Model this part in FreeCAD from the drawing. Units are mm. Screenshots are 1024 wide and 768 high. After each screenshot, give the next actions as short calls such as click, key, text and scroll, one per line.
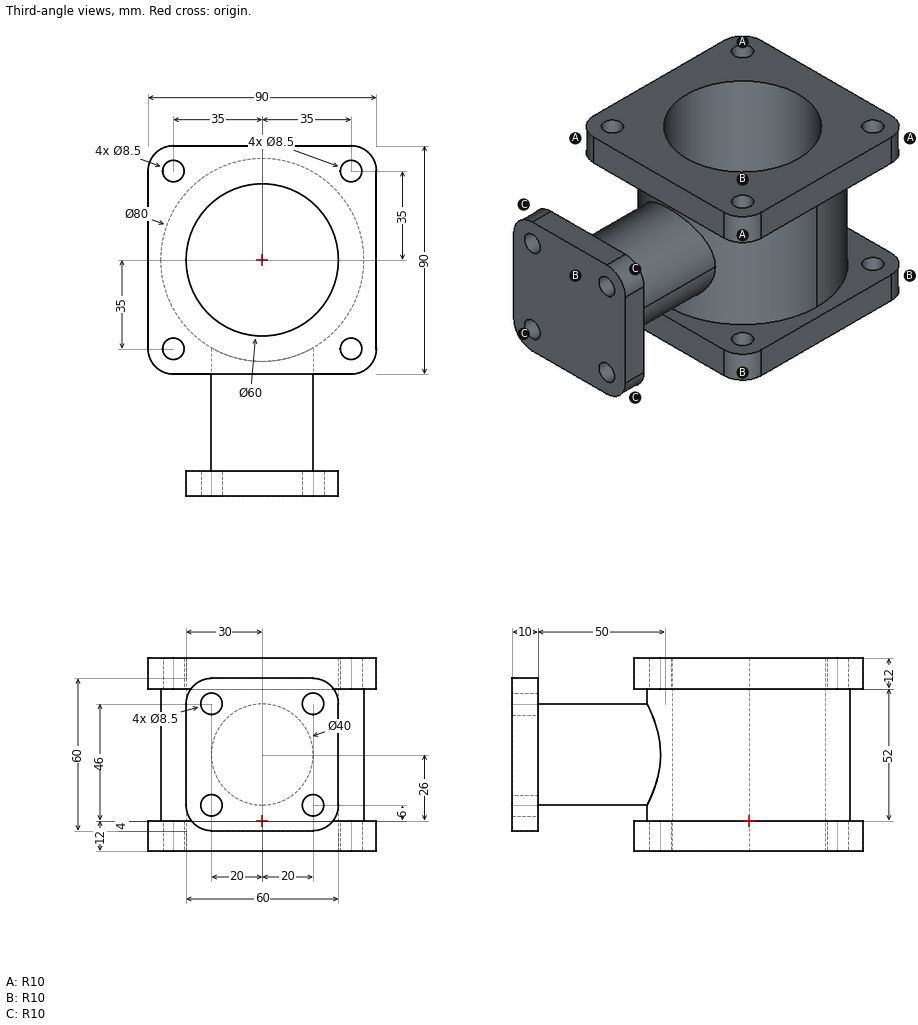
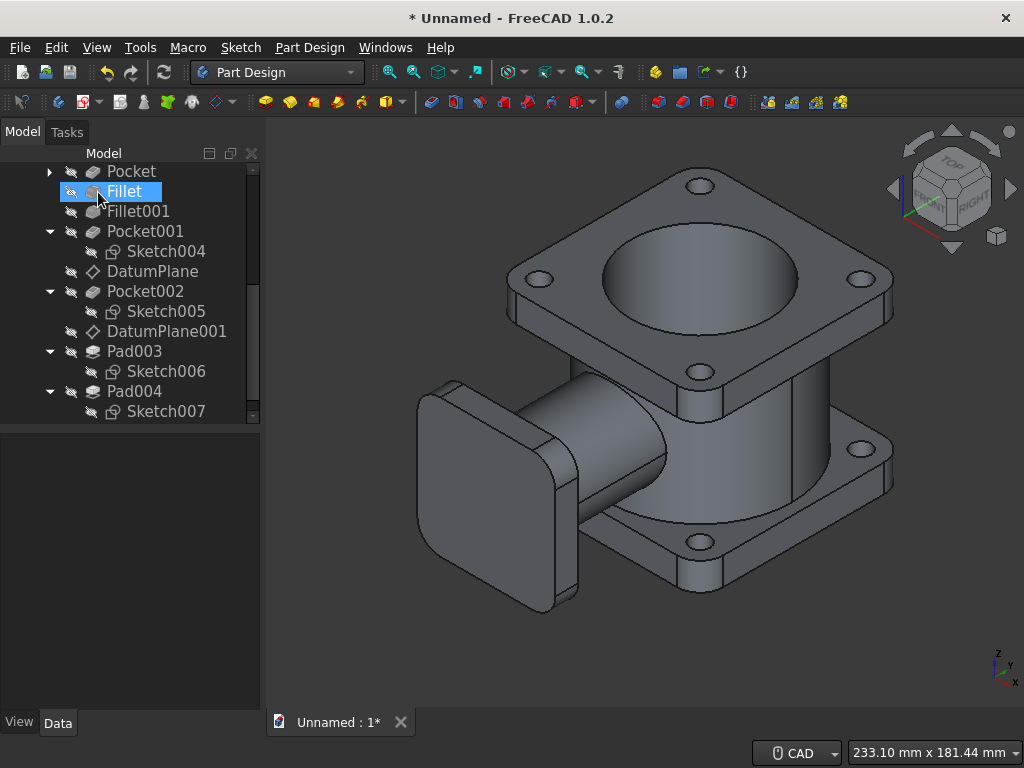
click(486, 503)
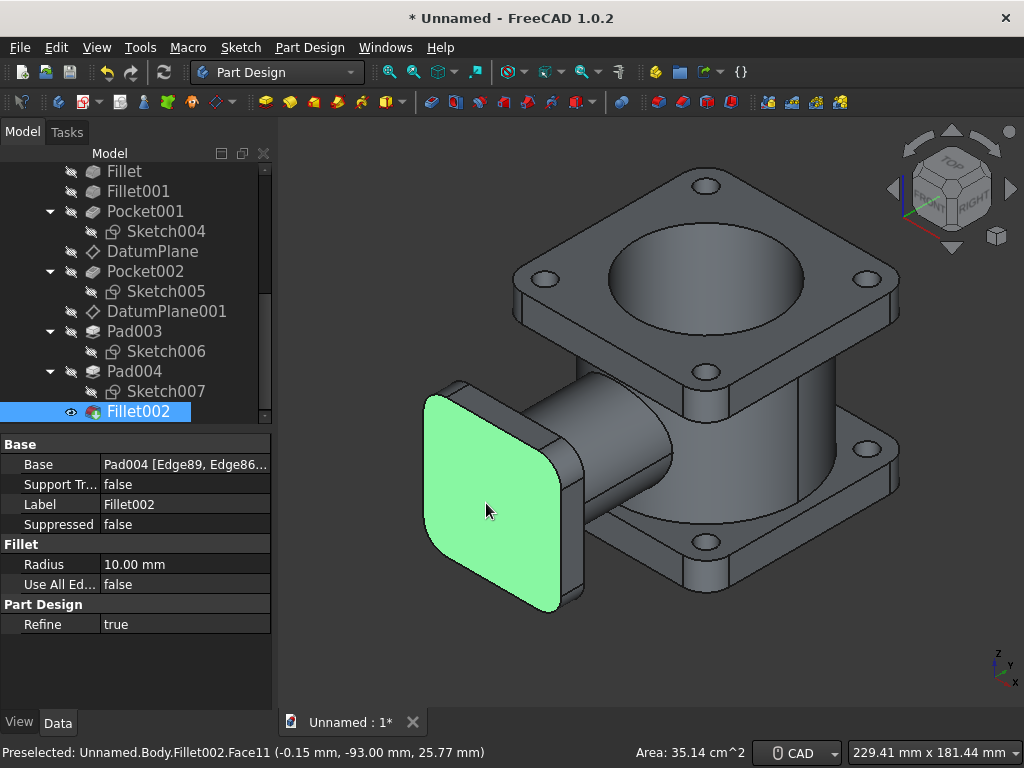
click(84, 102)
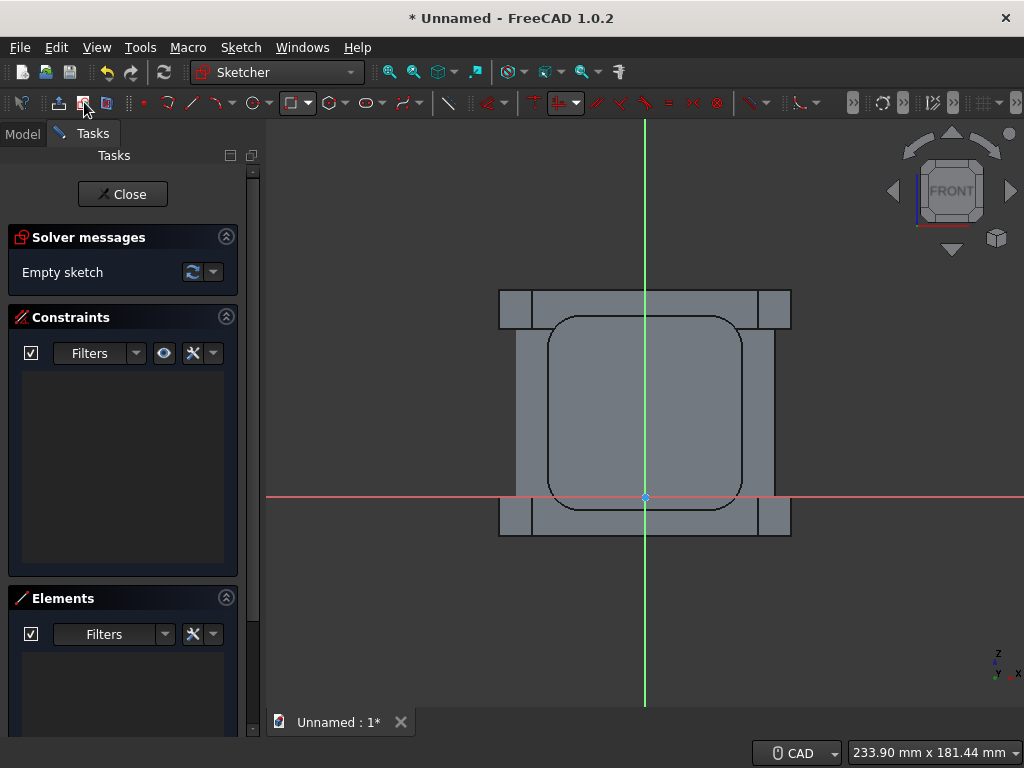
scroll(701, 418, up, 4)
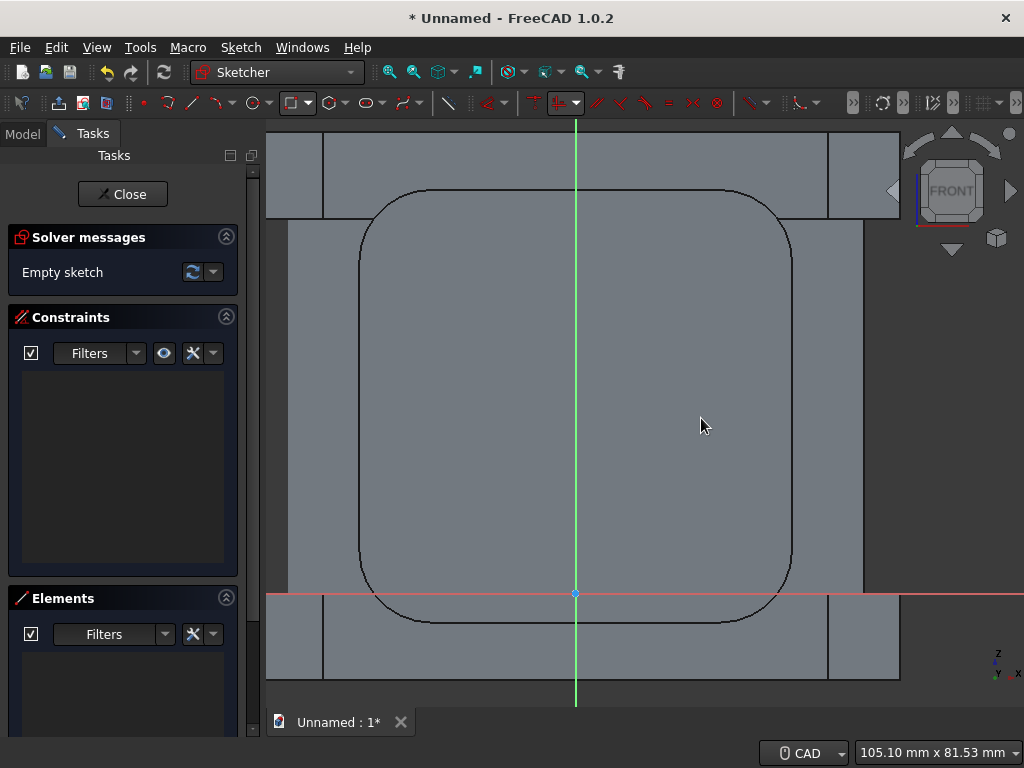
click(254, 104)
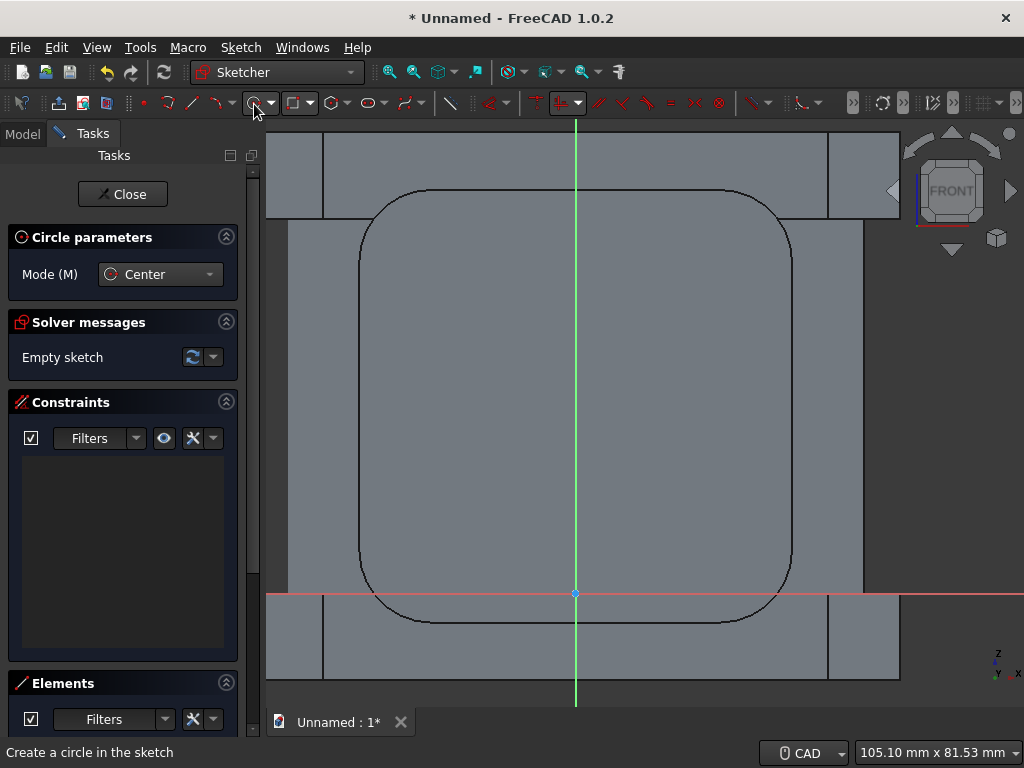
click(431, 262)
click(453, 240)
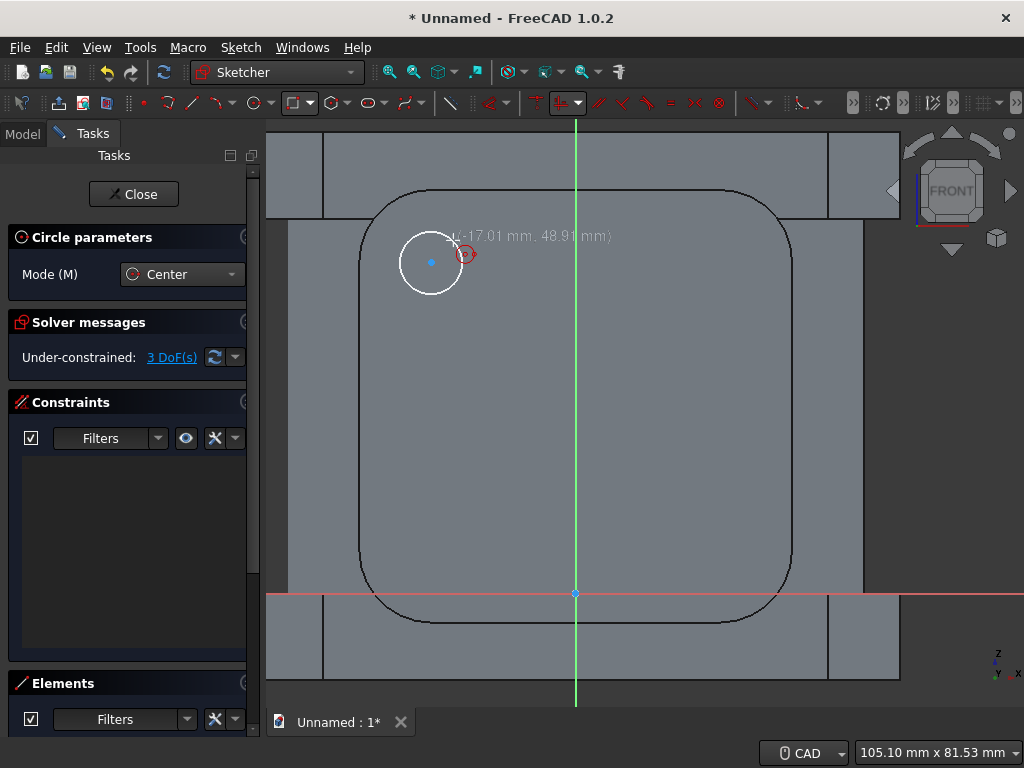
click(720, 262)
click(742, 240)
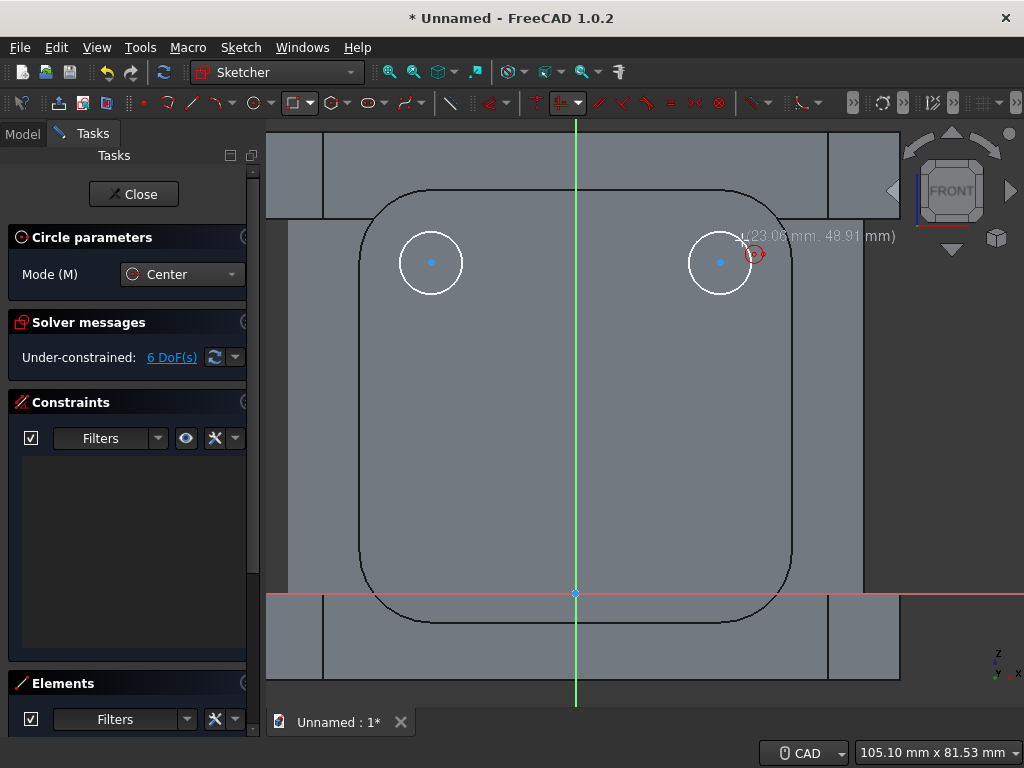
click(720, 550)
click(742, 529)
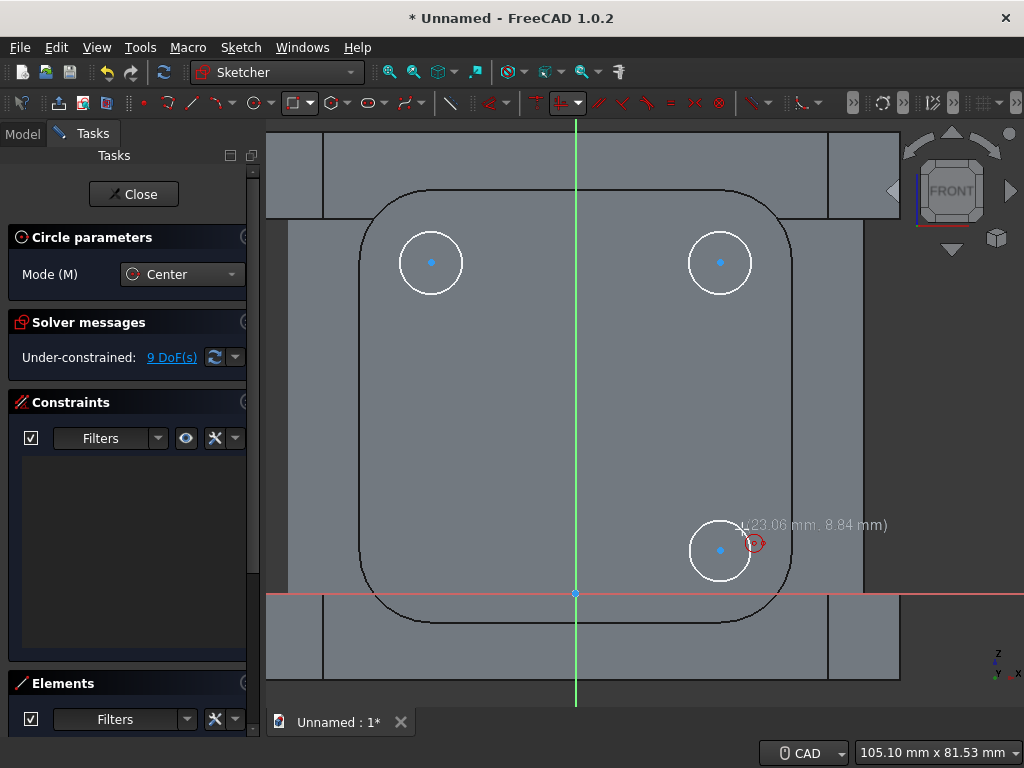
click(431, 550)
click(453, 529)
key(Escape)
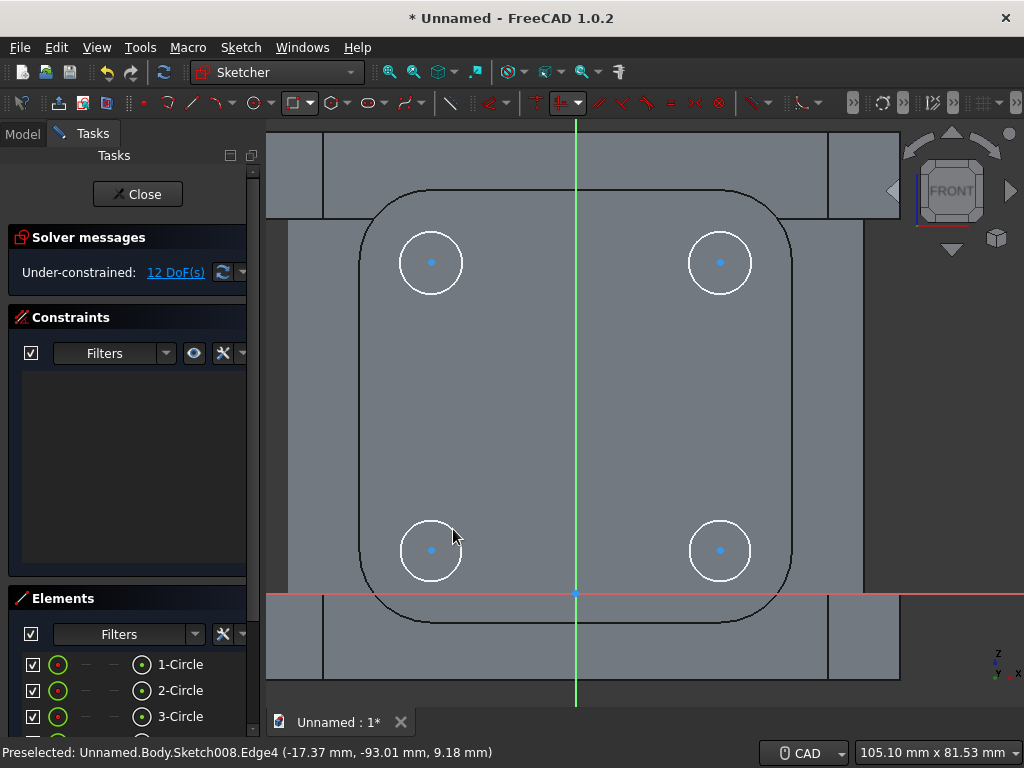
click(453, 241)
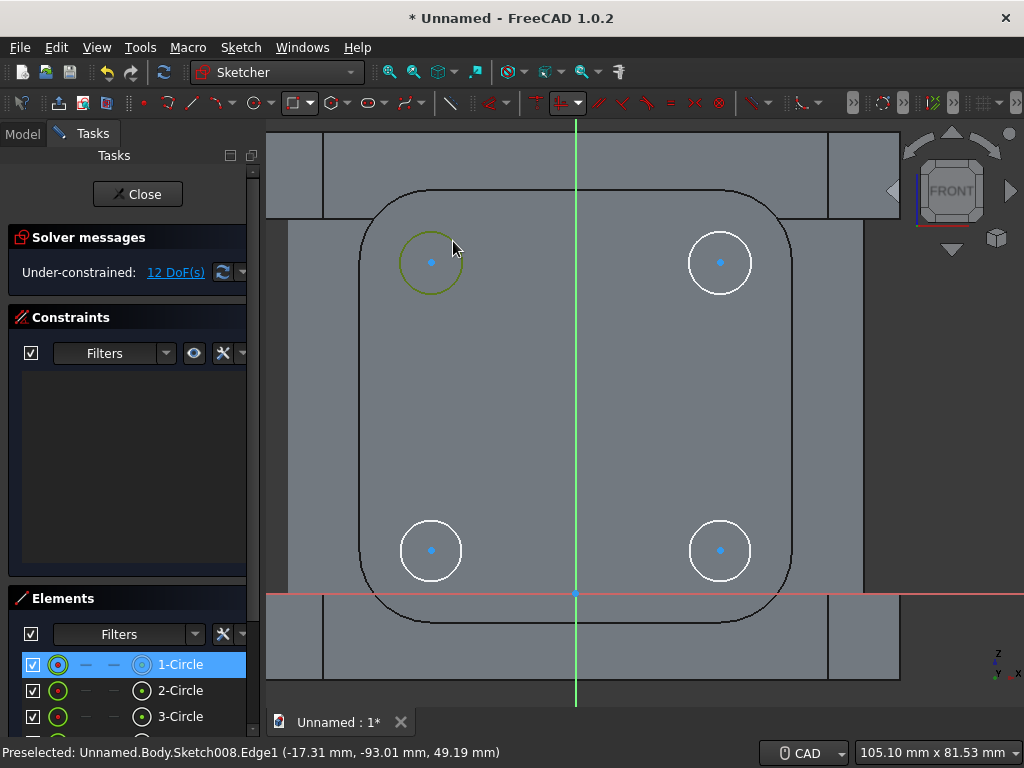
click(742, 241)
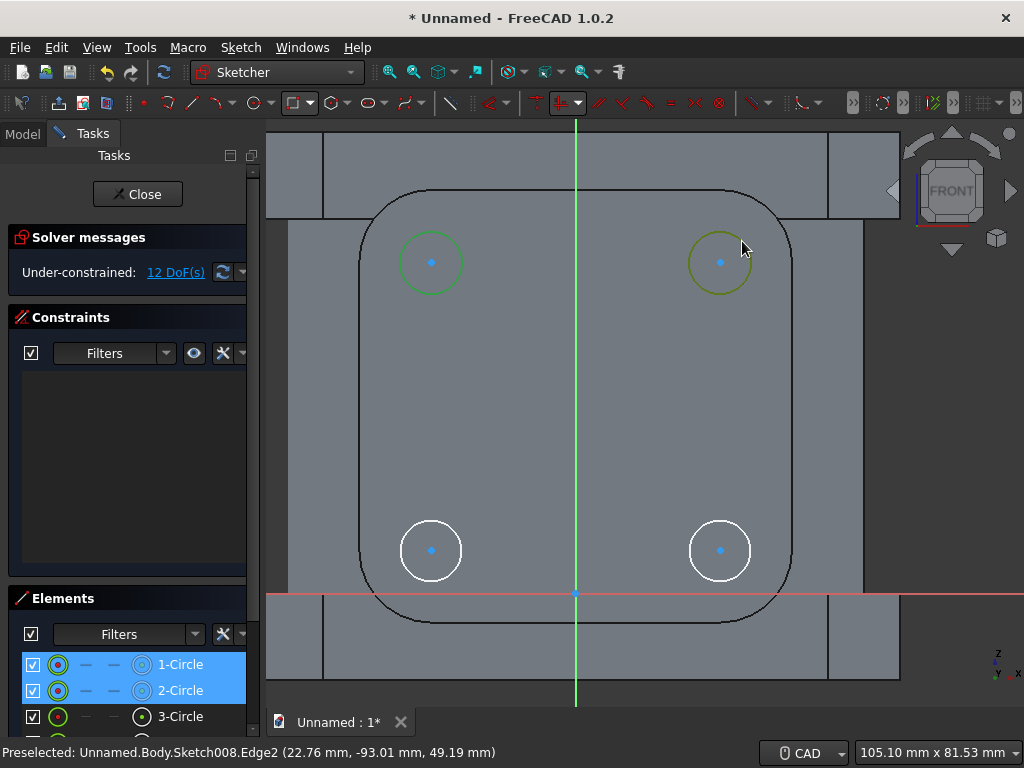
click(741, 529)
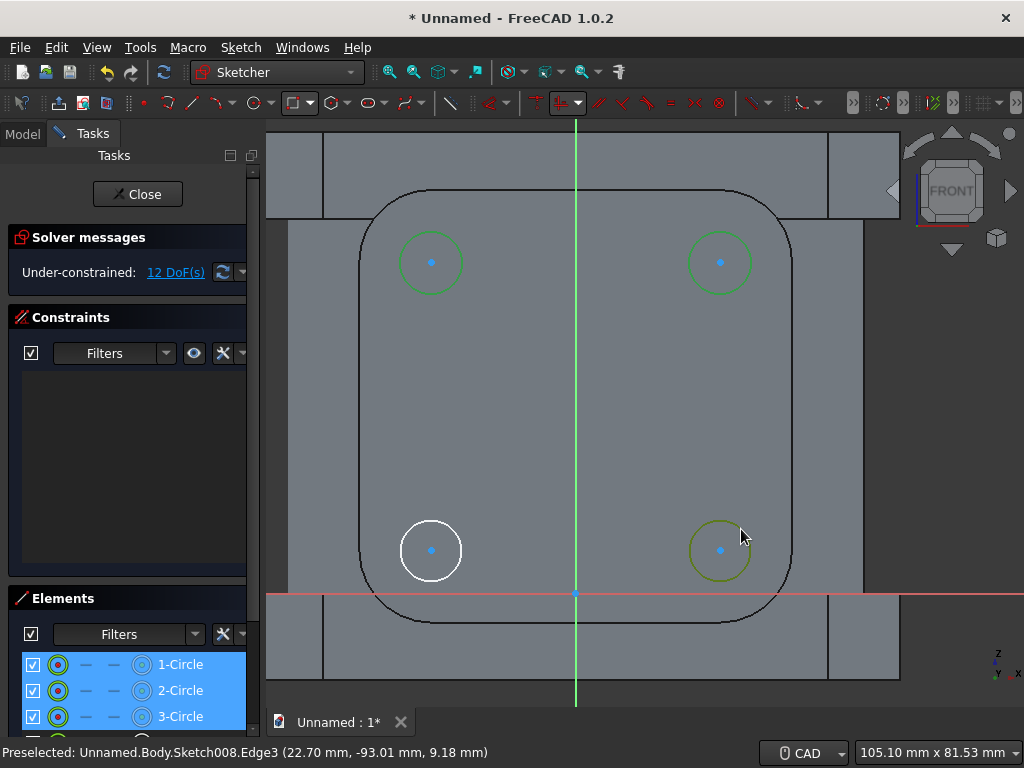
click(452, 529)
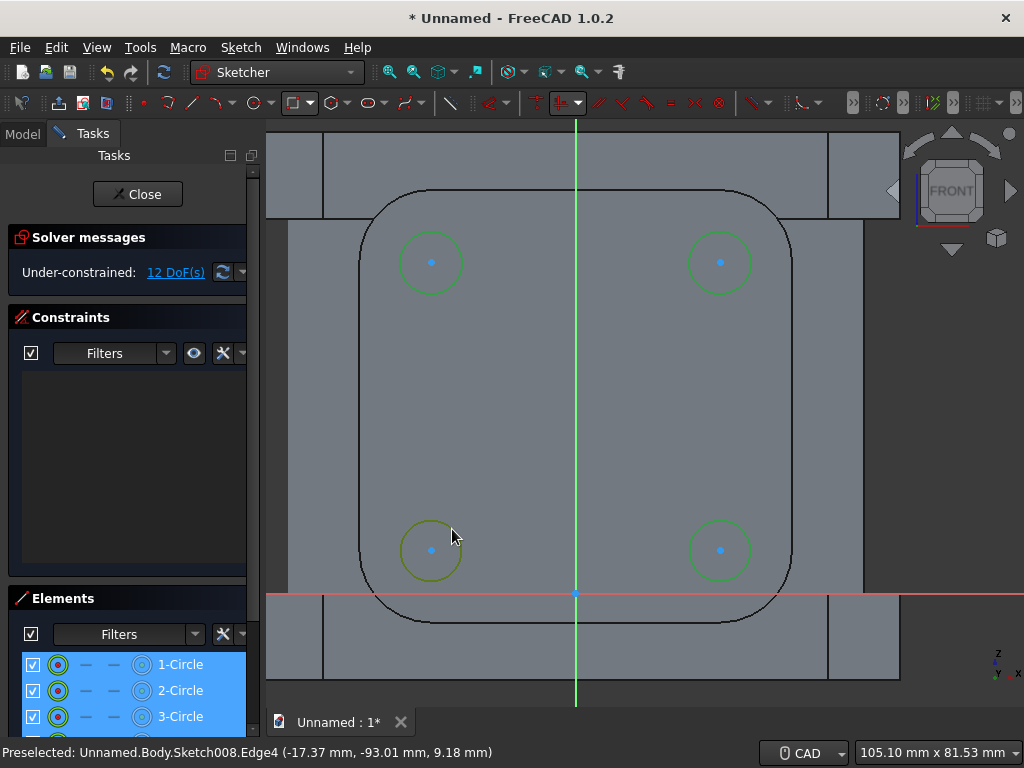
key(e)